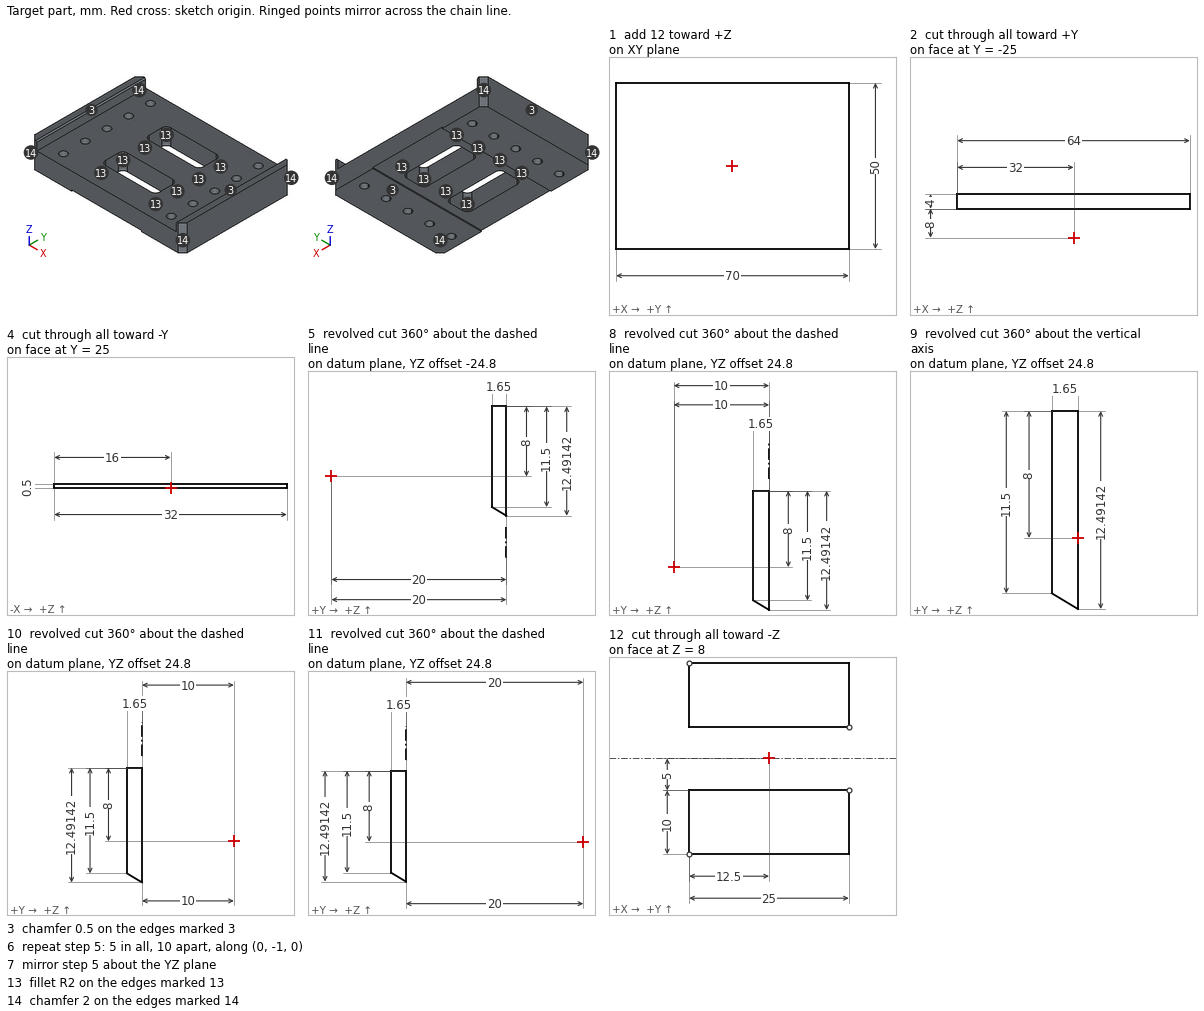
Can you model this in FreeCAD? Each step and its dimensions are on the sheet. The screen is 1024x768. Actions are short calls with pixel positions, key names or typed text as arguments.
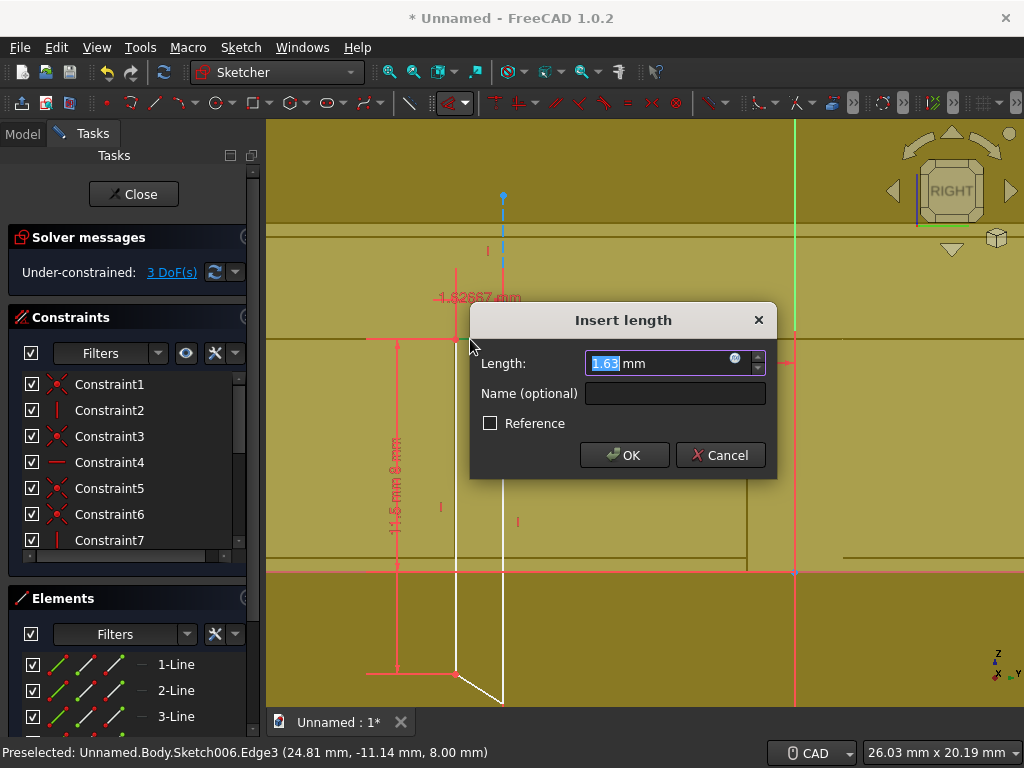
text(1.65)
key(Return)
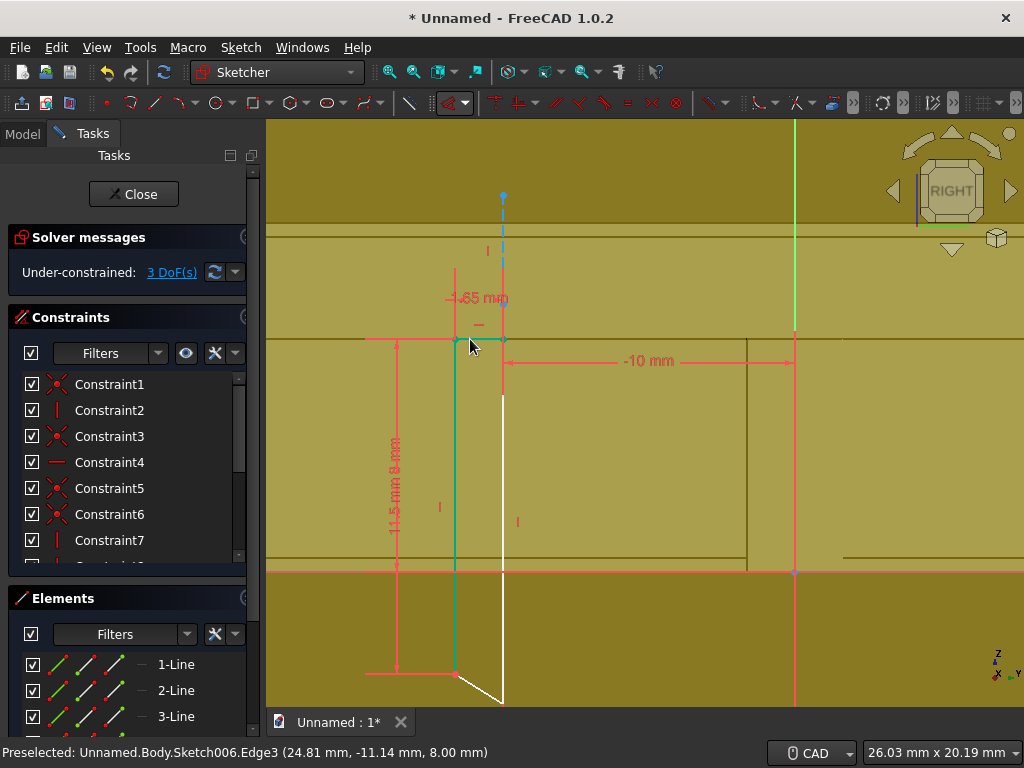
click(503, 449)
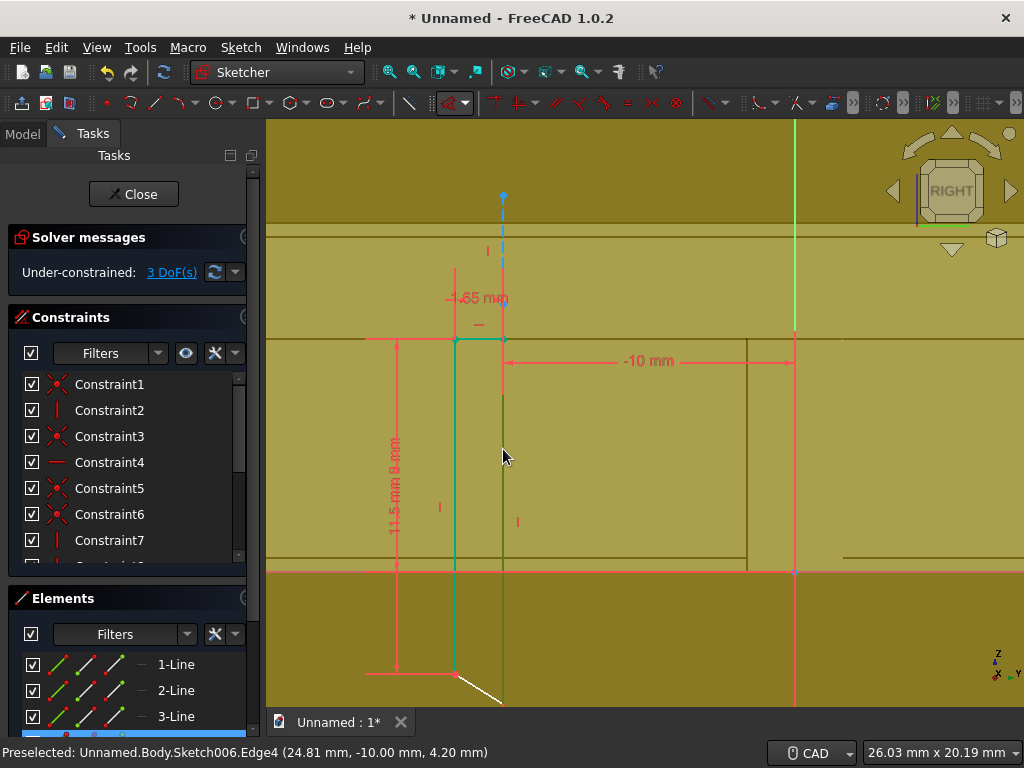
key(i)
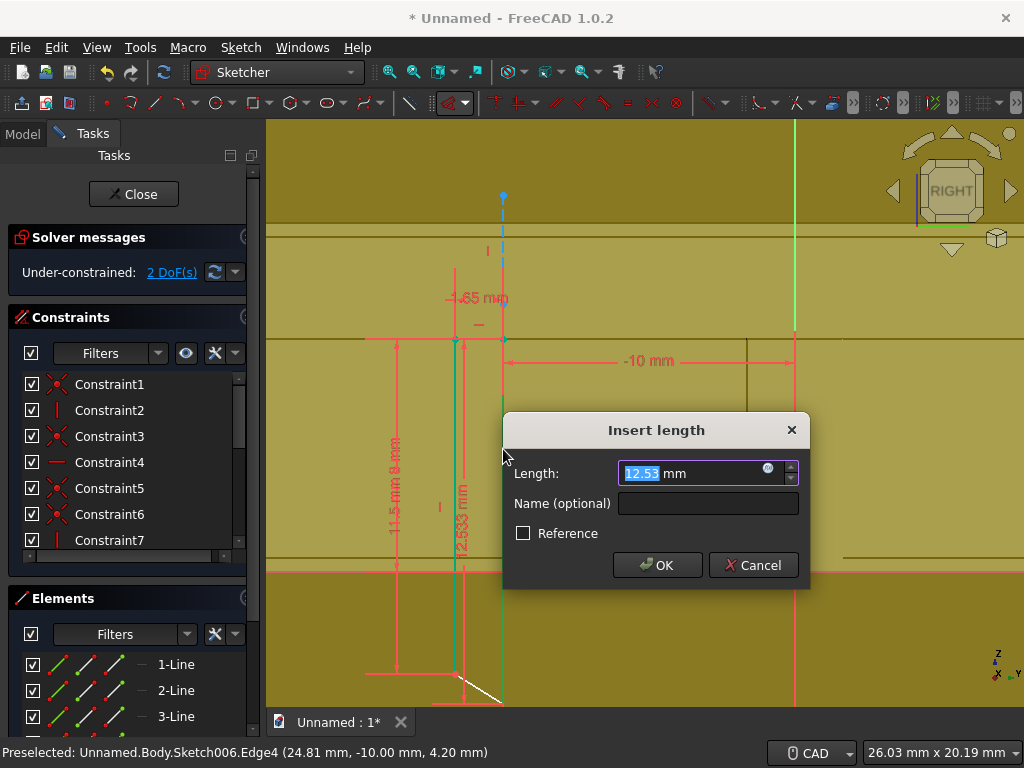
text(12.49142)
key(Return)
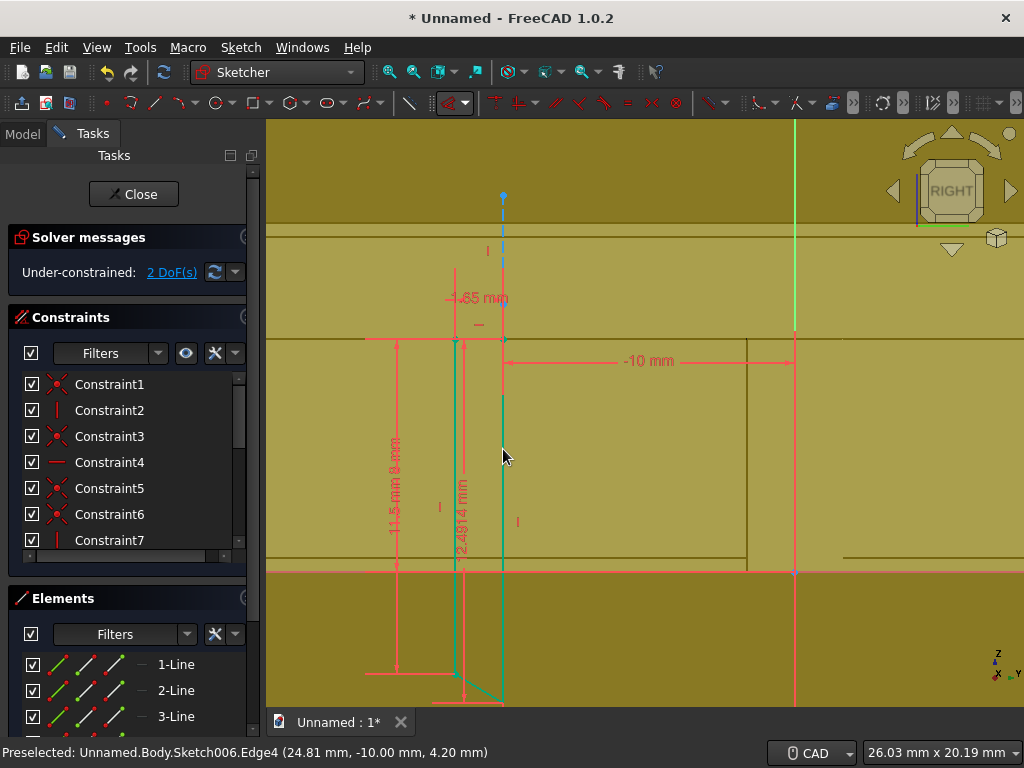
click(134, 194)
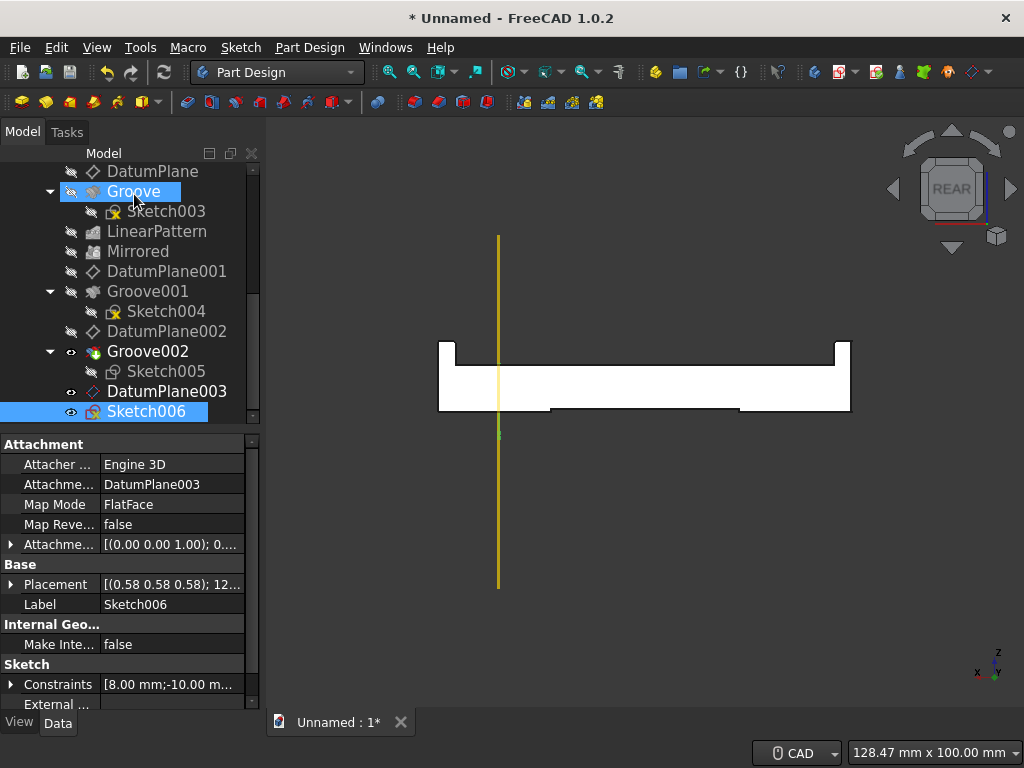
click(236, 102)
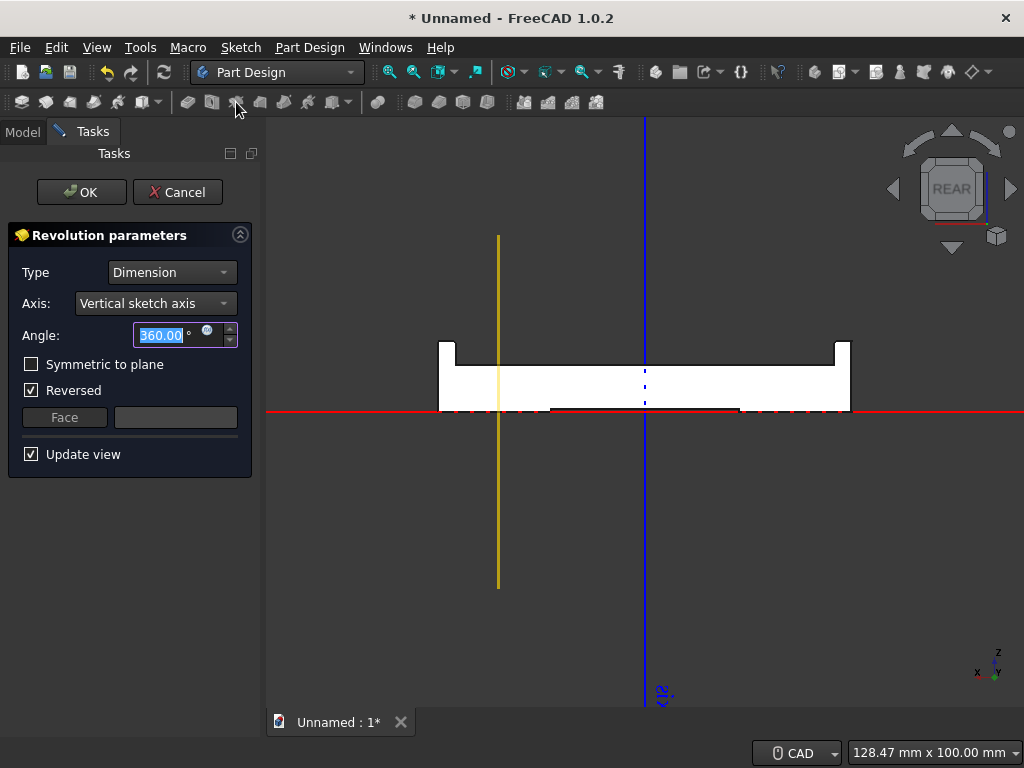
click(156, 304)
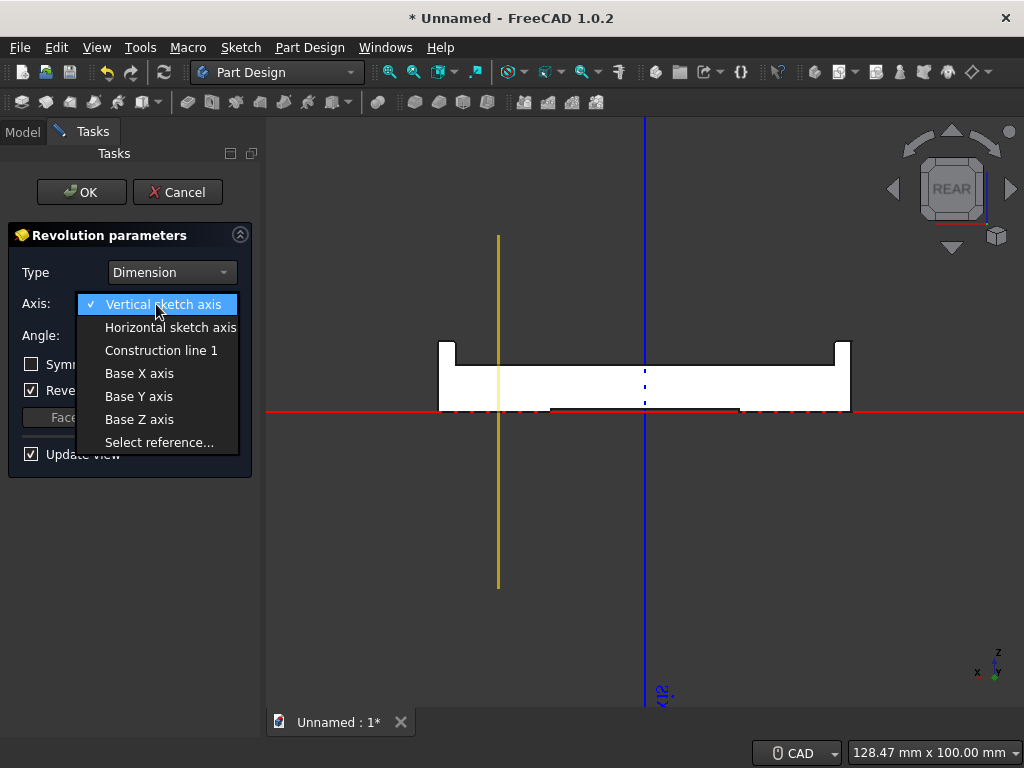
click(156, 350)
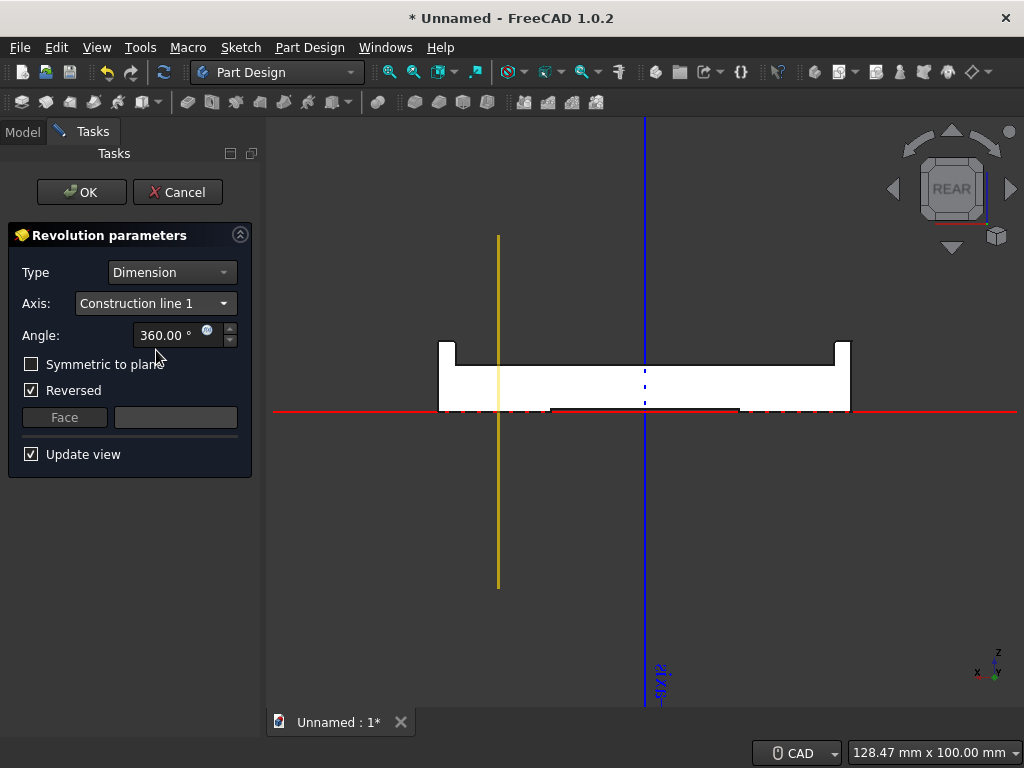
click(82, 192)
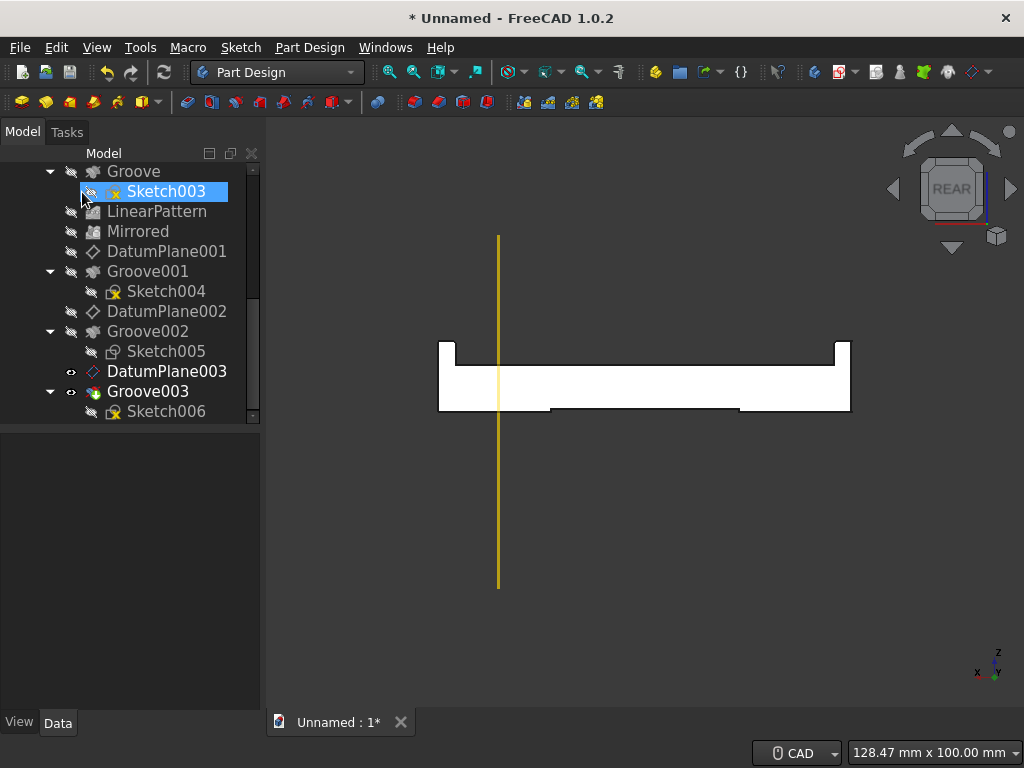
click(116, 372)
key(space)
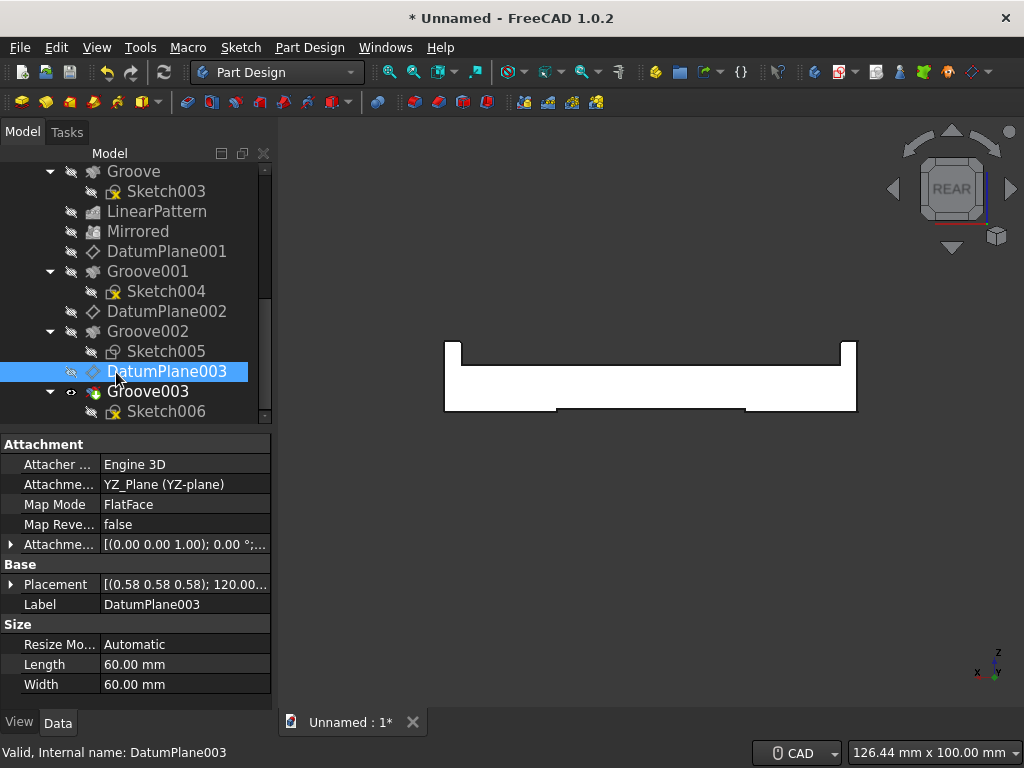
scroll(140, 287, down, 3)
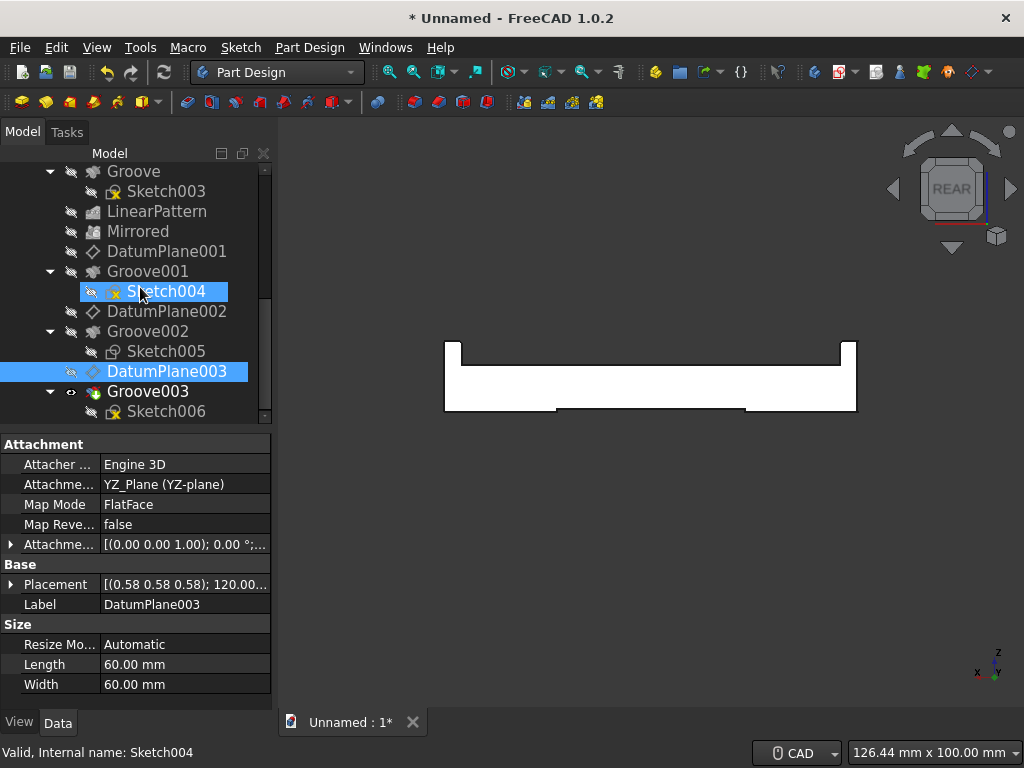
scroll(140, 287, up, 15)